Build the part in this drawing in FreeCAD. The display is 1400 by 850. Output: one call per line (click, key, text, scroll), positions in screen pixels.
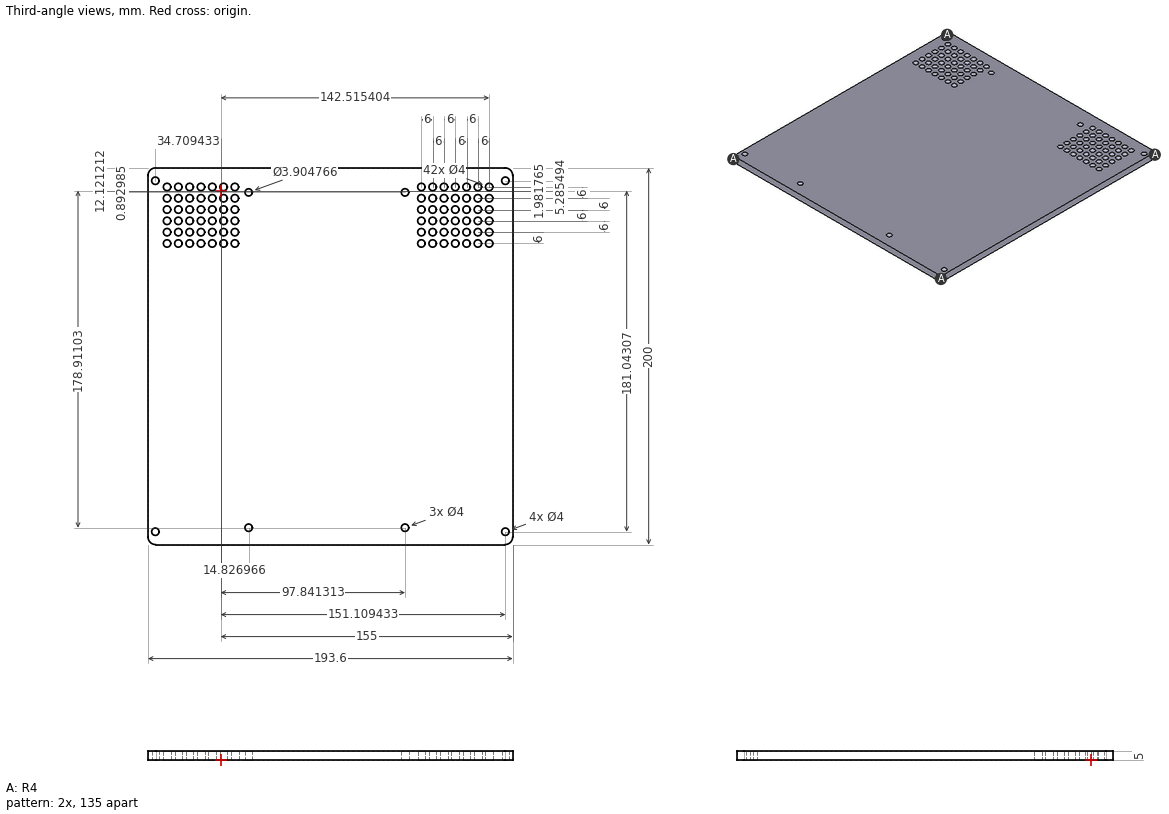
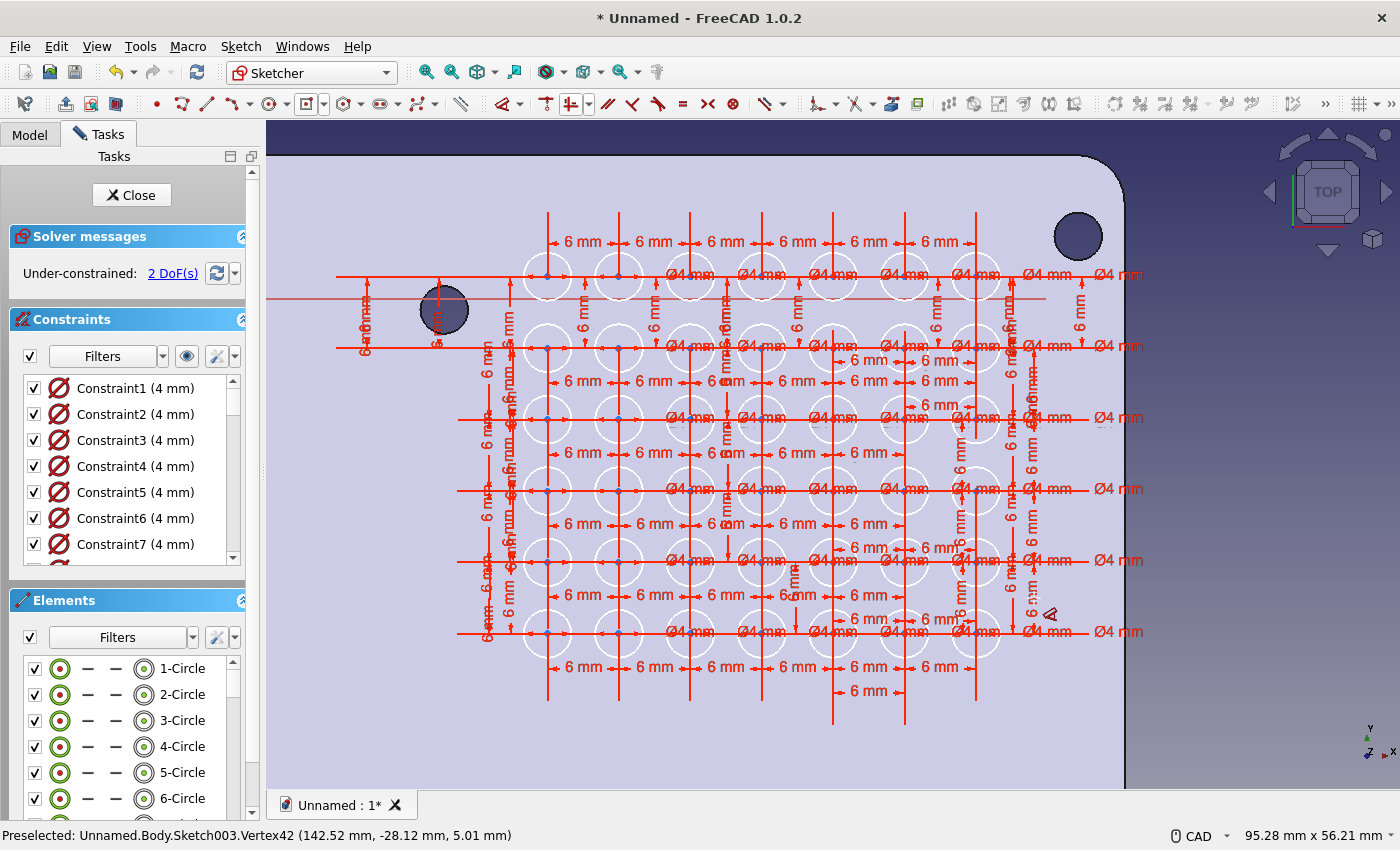
scroll(976, 277, up, 3)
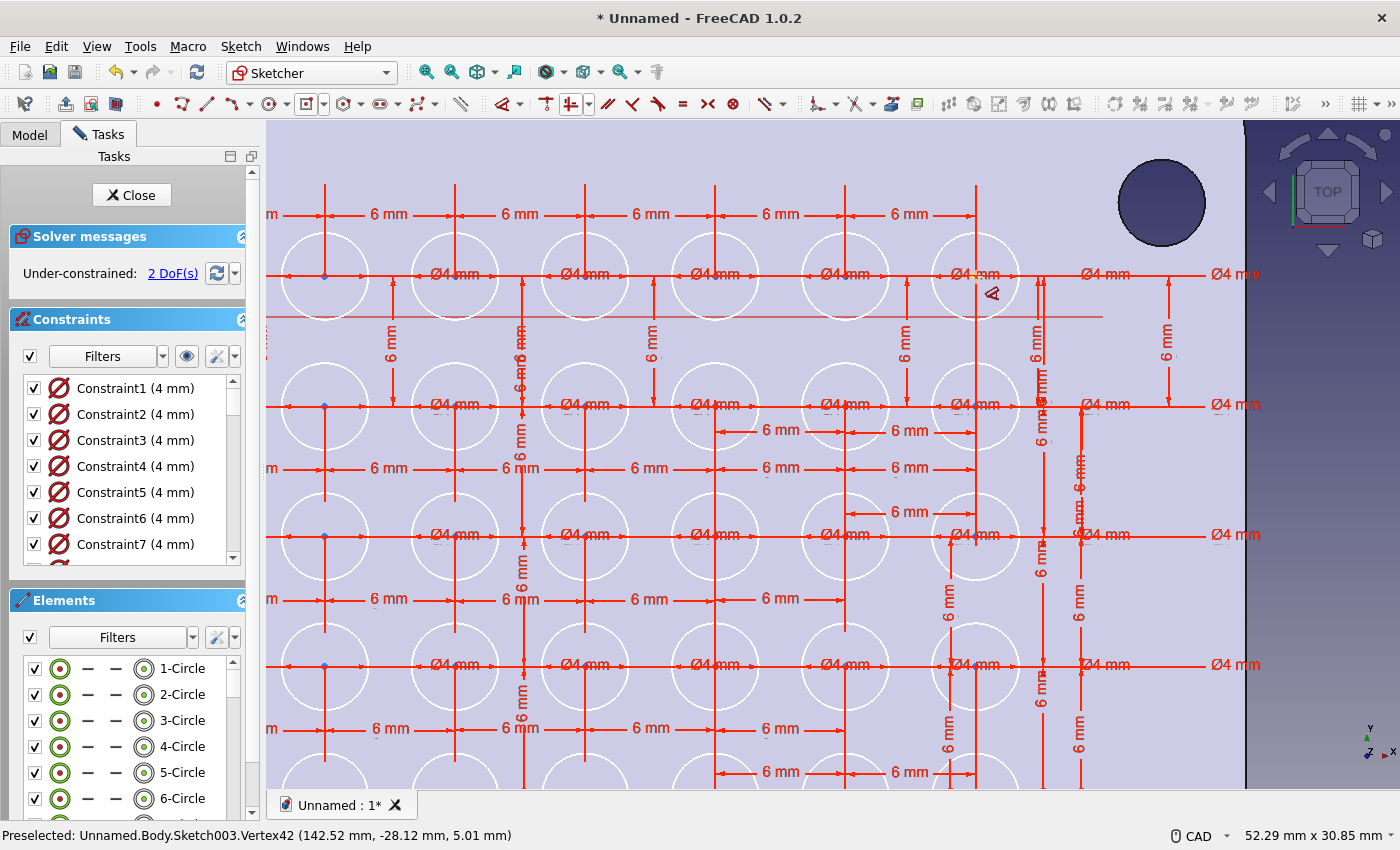
click(976, 276)
click(1034, 297)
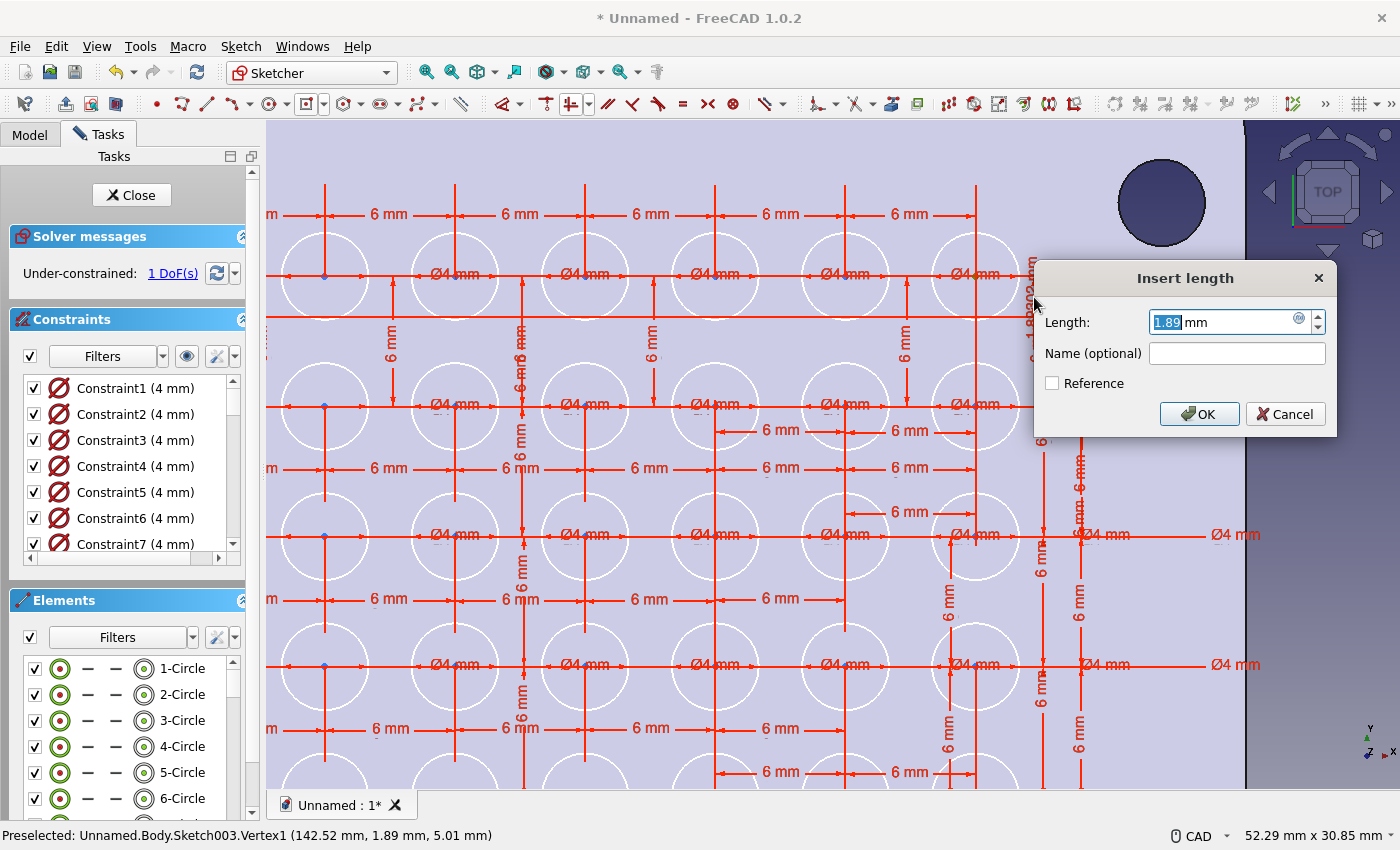
text(1.981765)
key(Return)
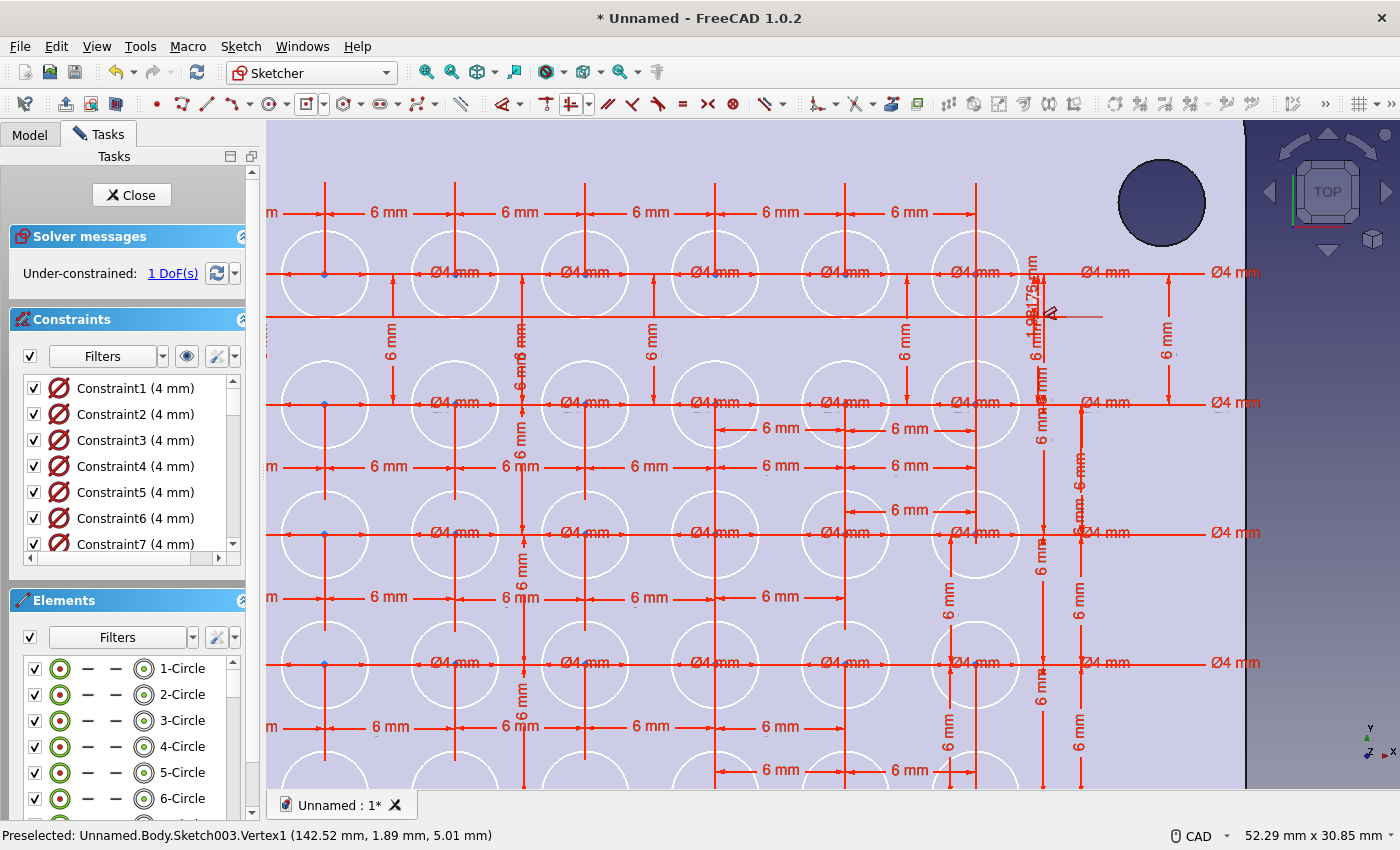
click(976, 274)
click(635, 240)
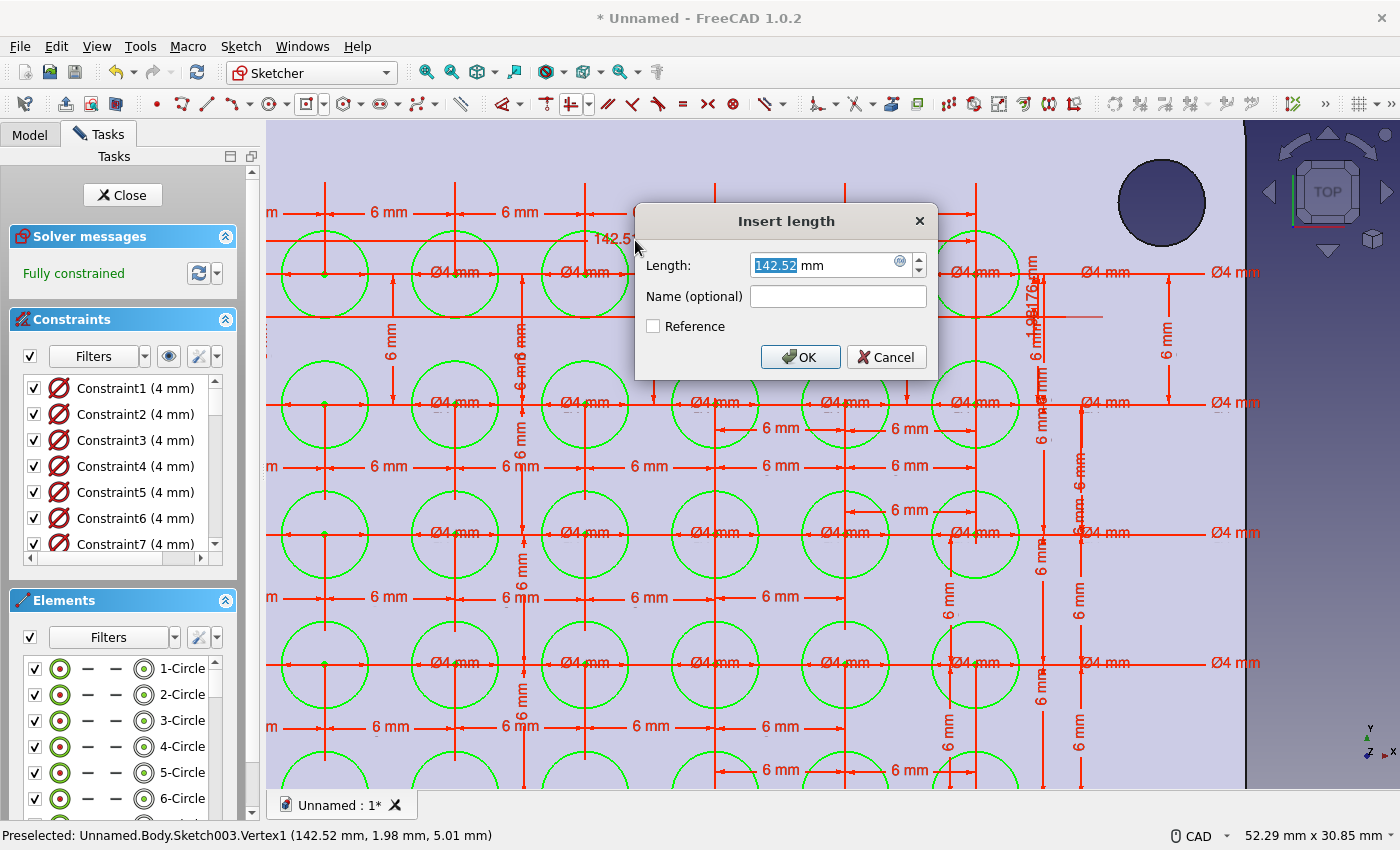
text(142.515404)
key(Return)
key(Escape)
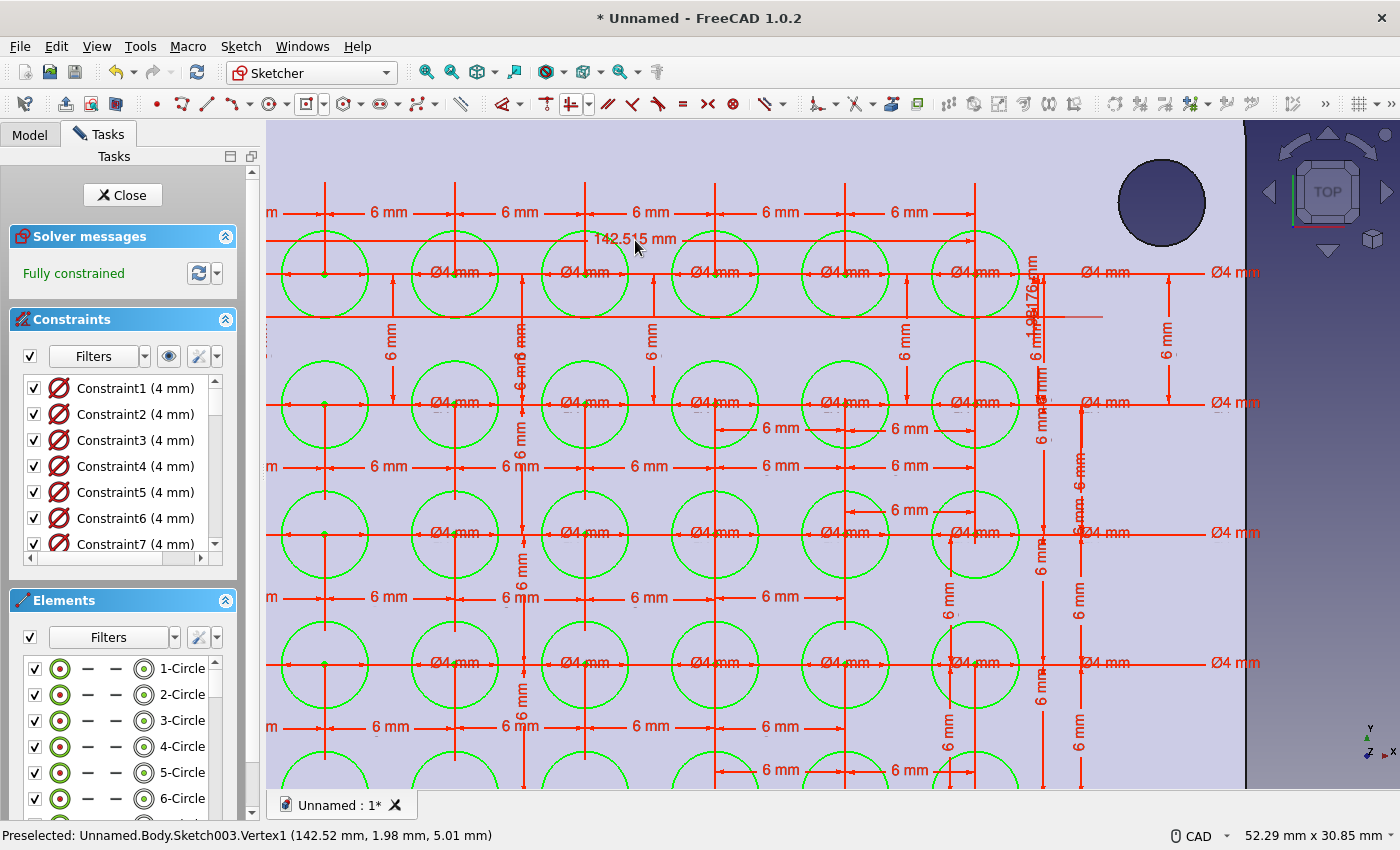
click(123, 195)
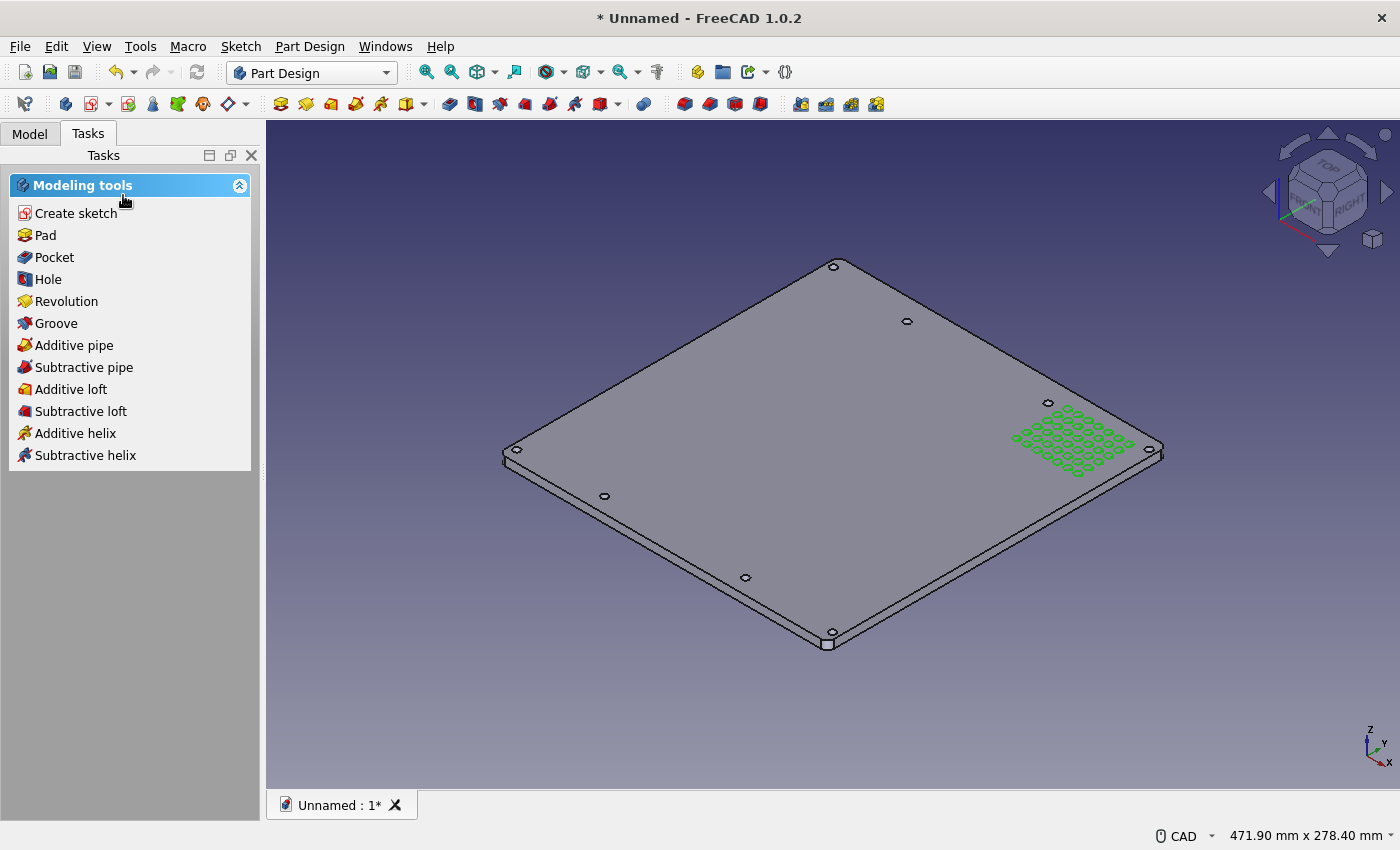
click(450, 104)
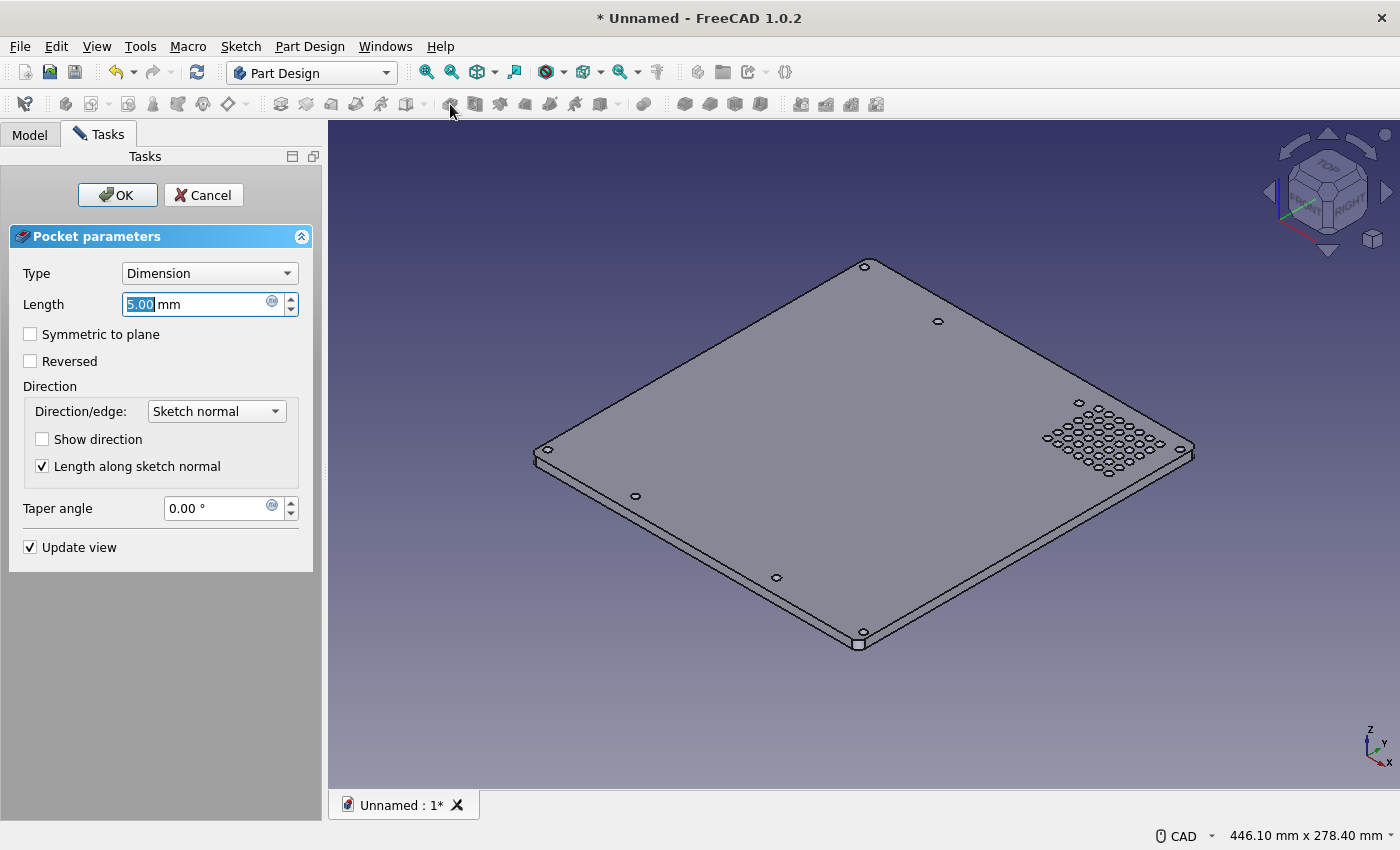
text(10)
key(Tab)